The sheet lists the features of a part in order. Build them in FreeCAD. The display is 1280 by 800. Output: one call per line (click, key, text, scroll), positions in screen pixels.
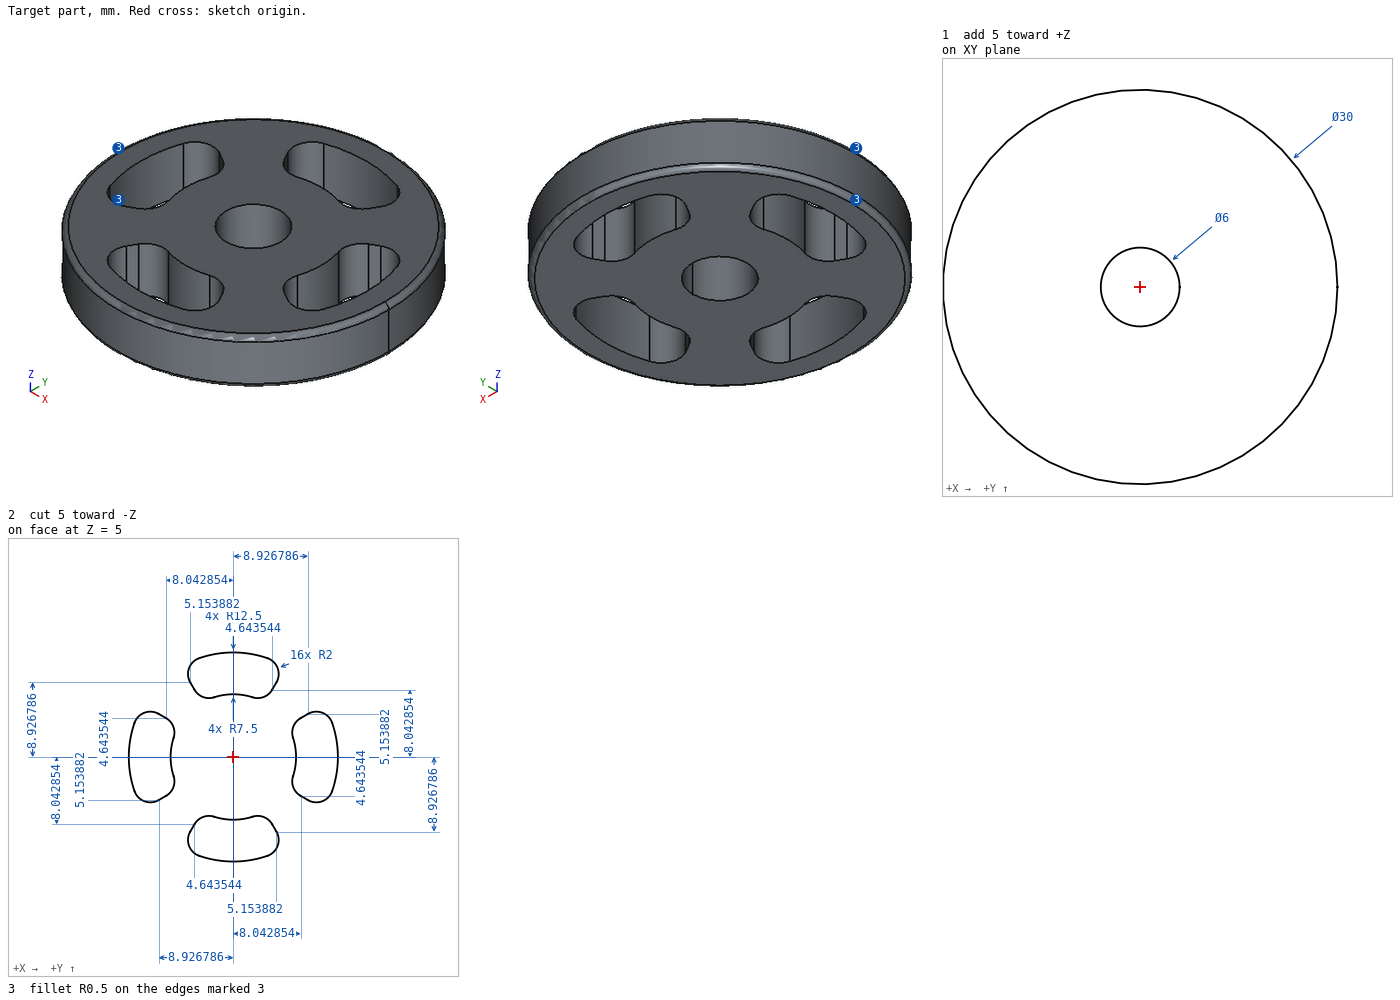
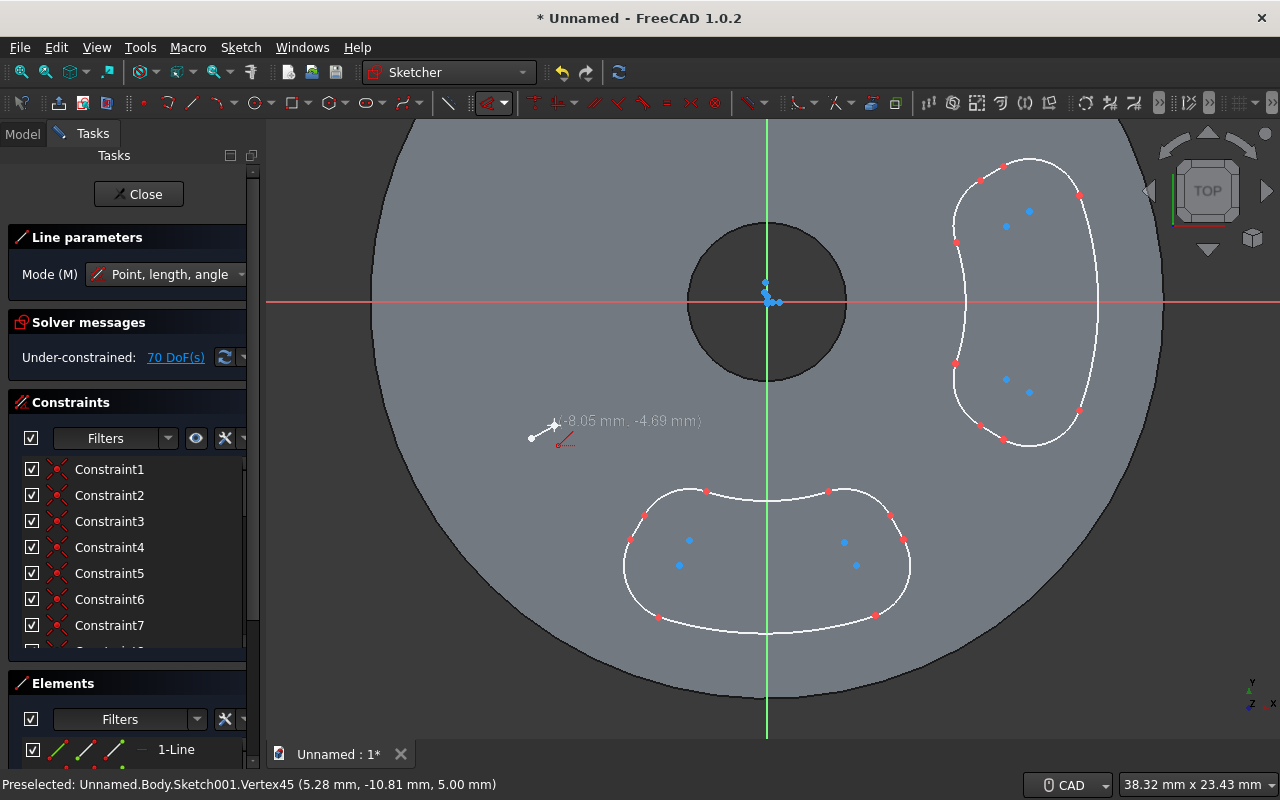
click(554, 179)
click(531, 166)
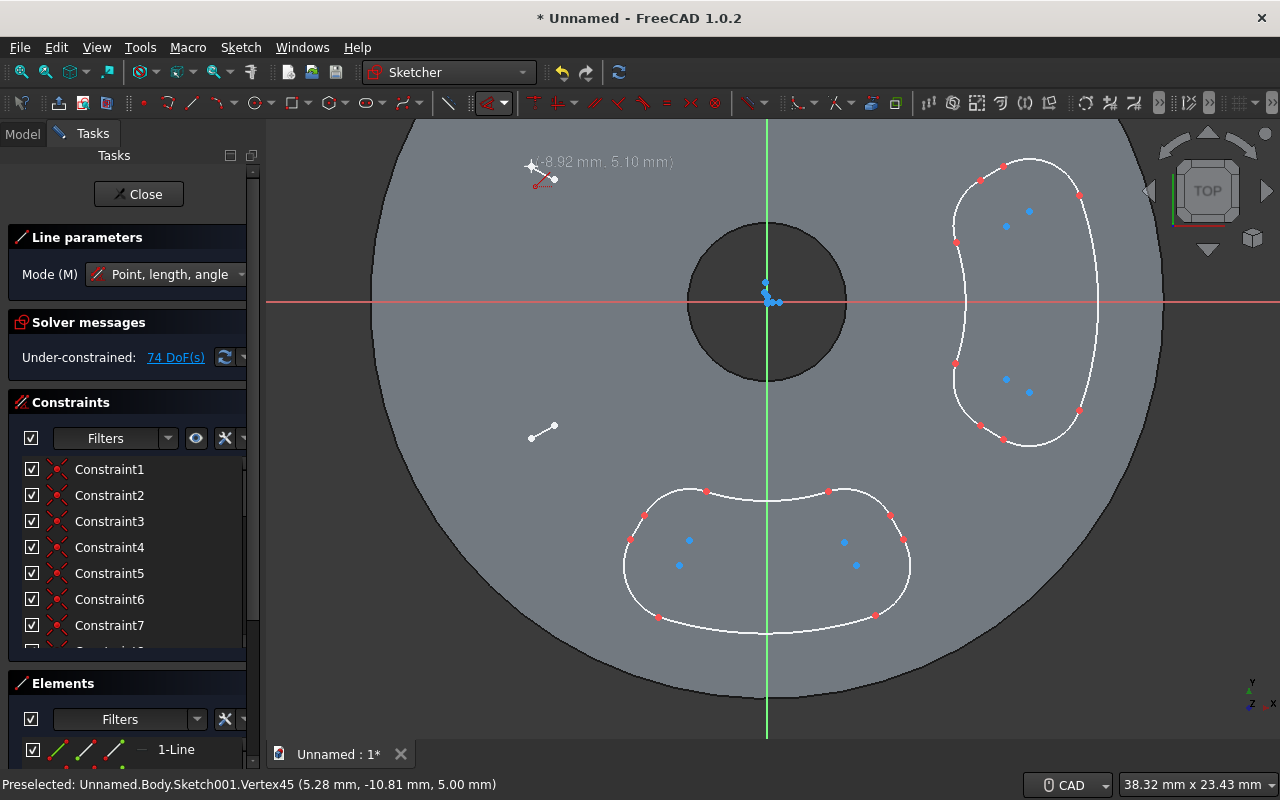
click(218, 104)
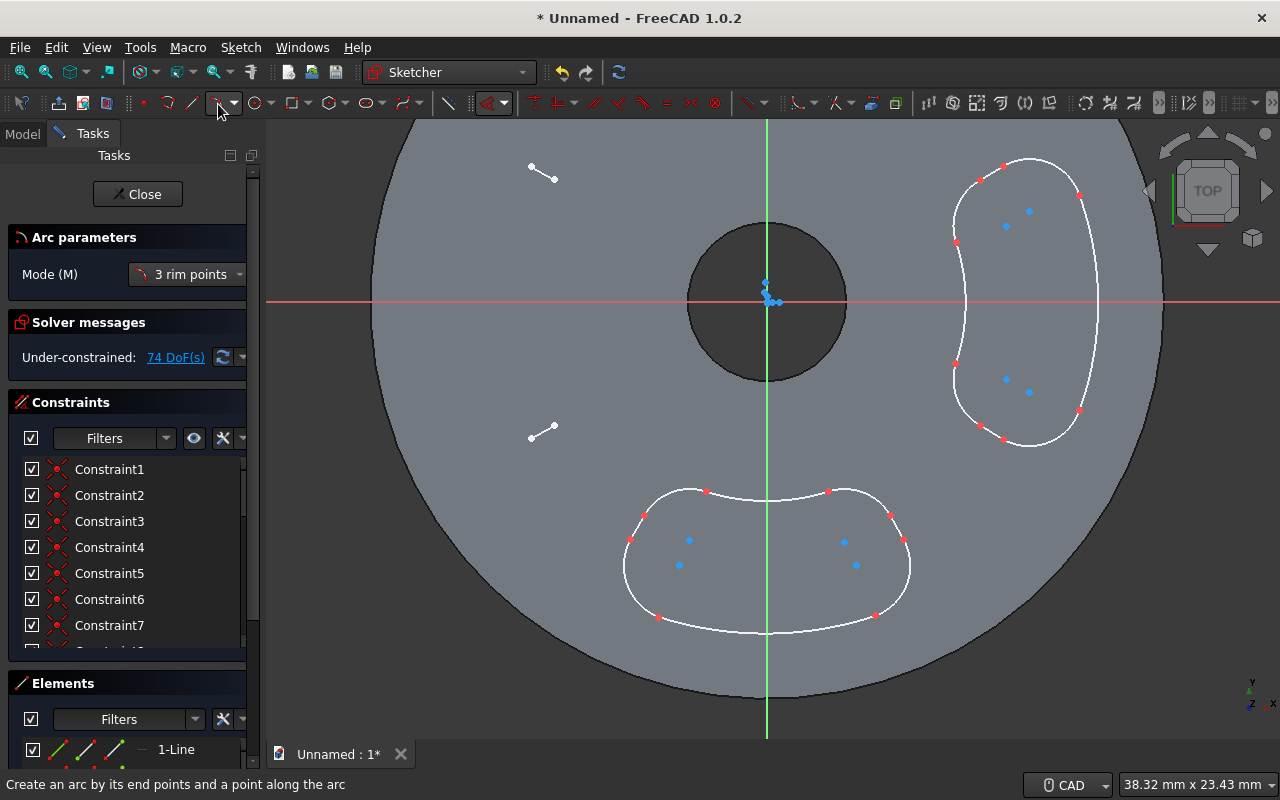
click(554, 426)
click(578, 363)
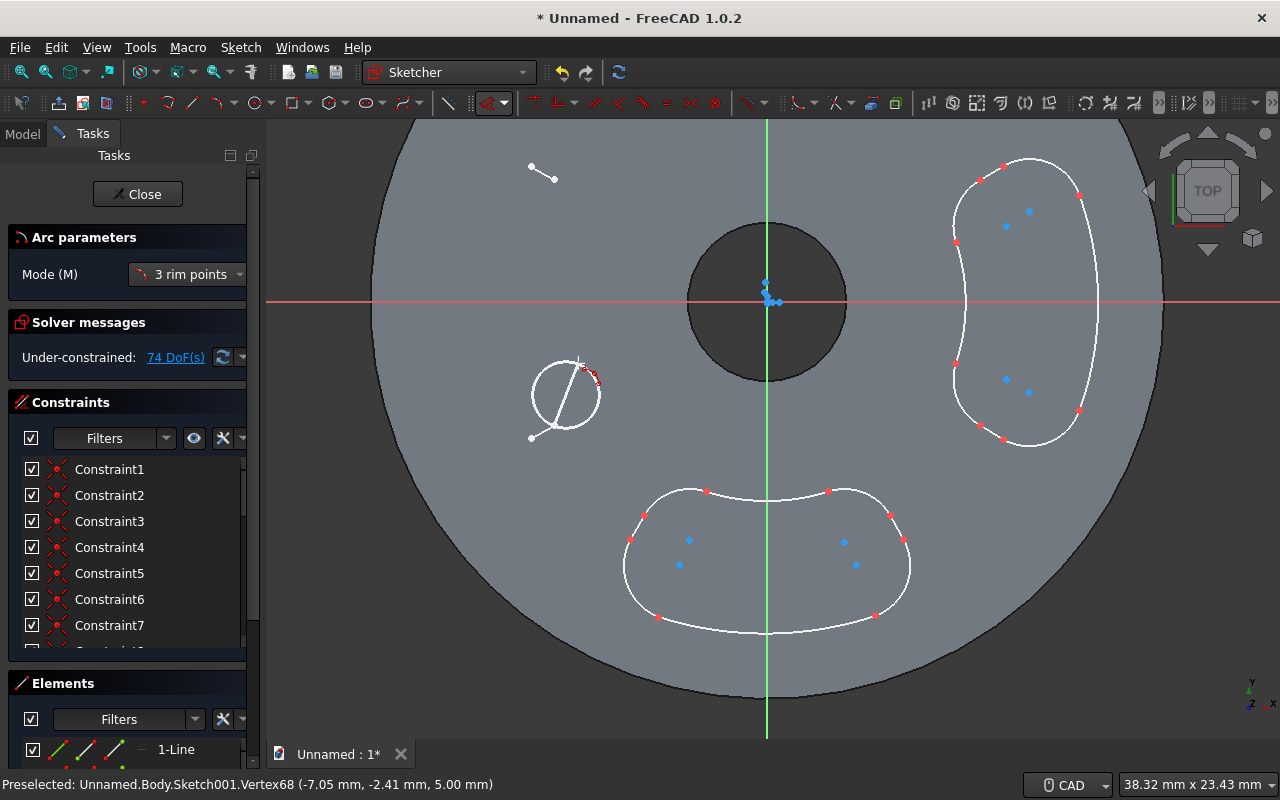
scroll(577, 398, up, 2)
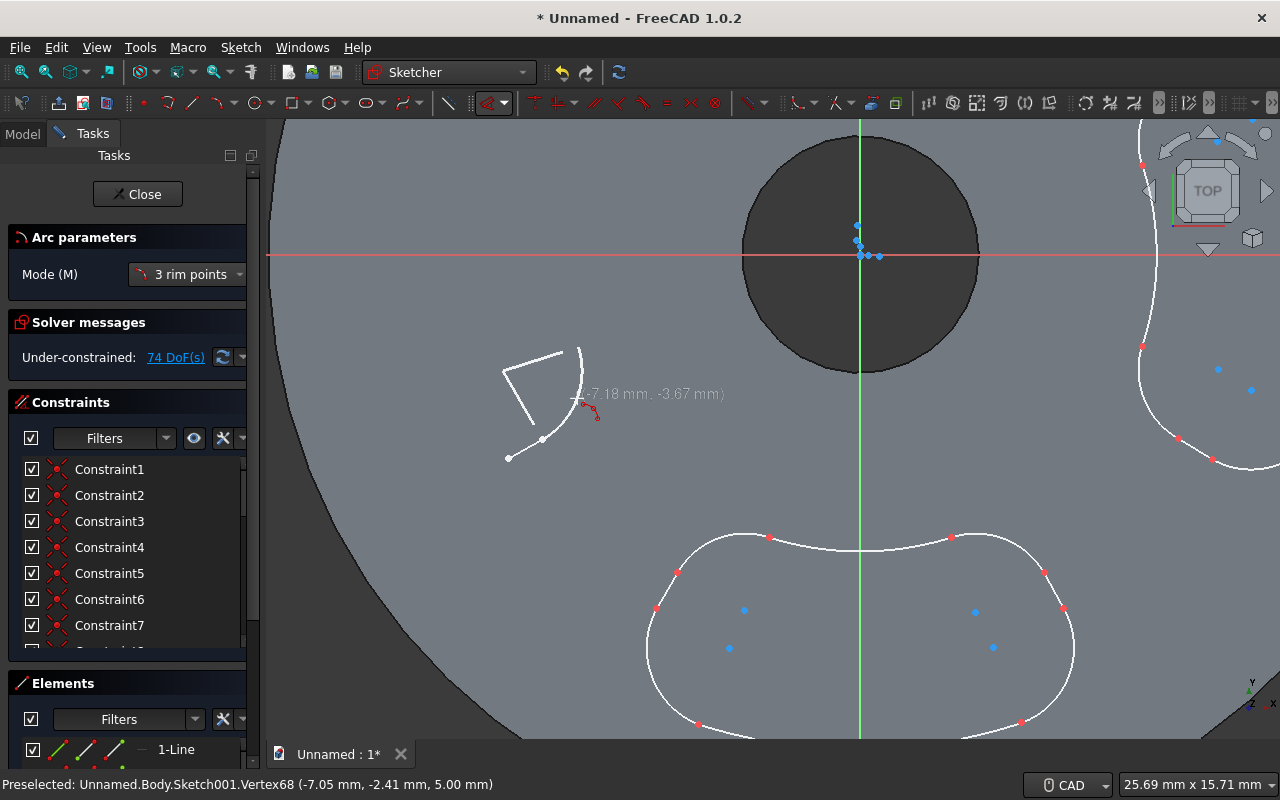
click(577, 398)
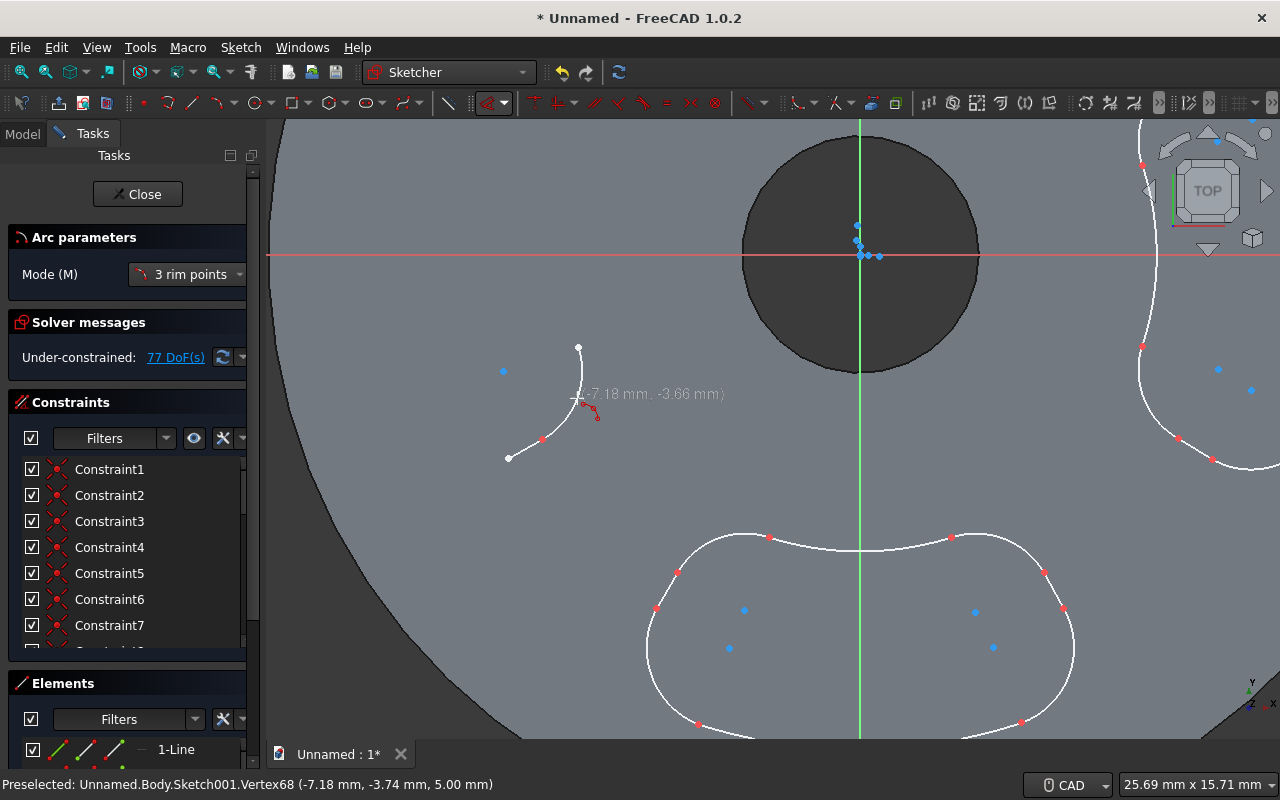
click(578, 347)
click(579, 164)
click(565, 236)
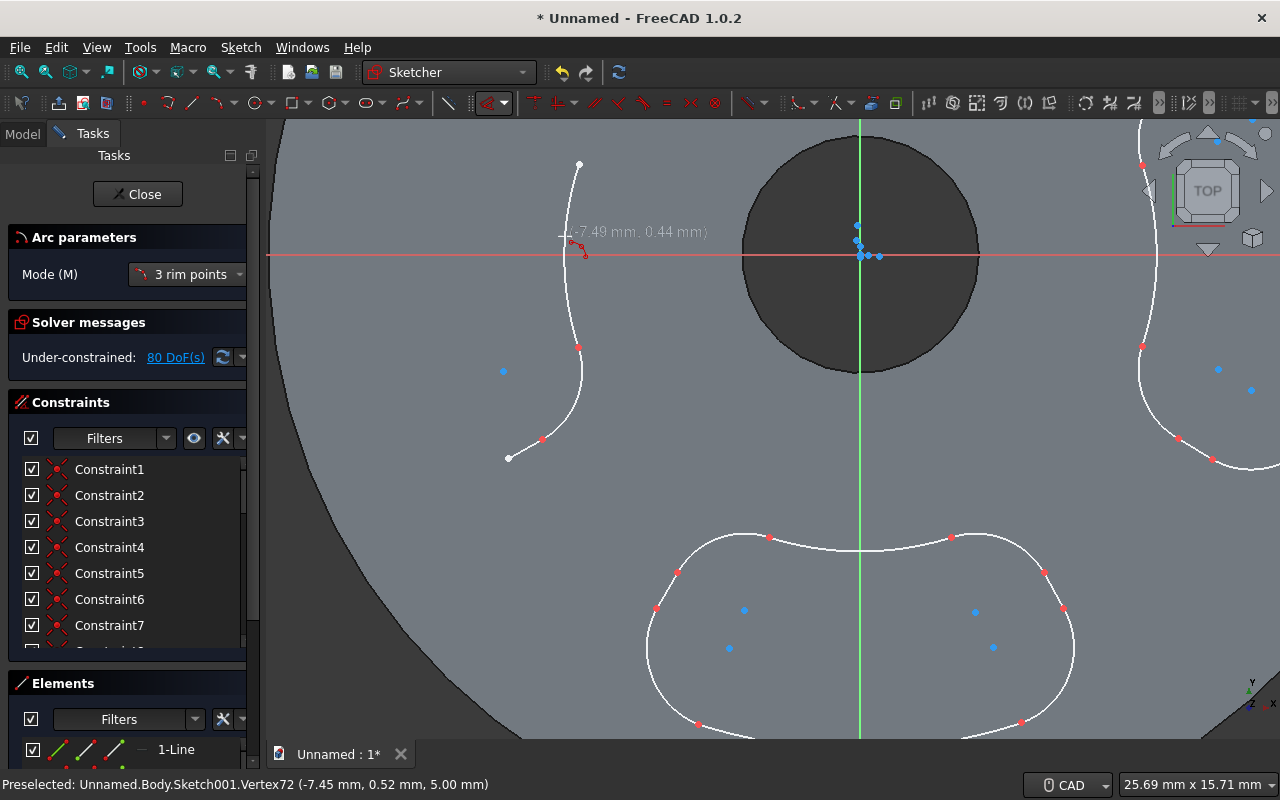
click(579, 165)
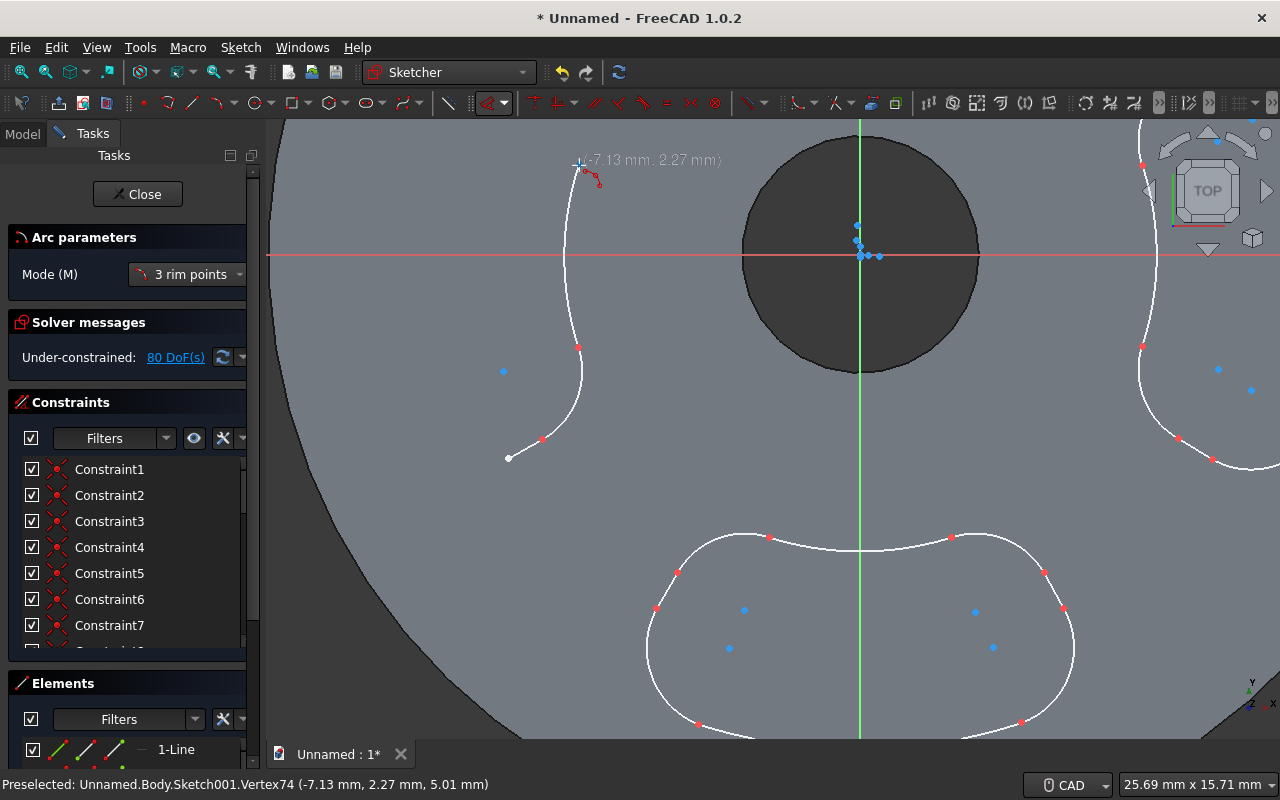
scroll(614, 531, down, 5)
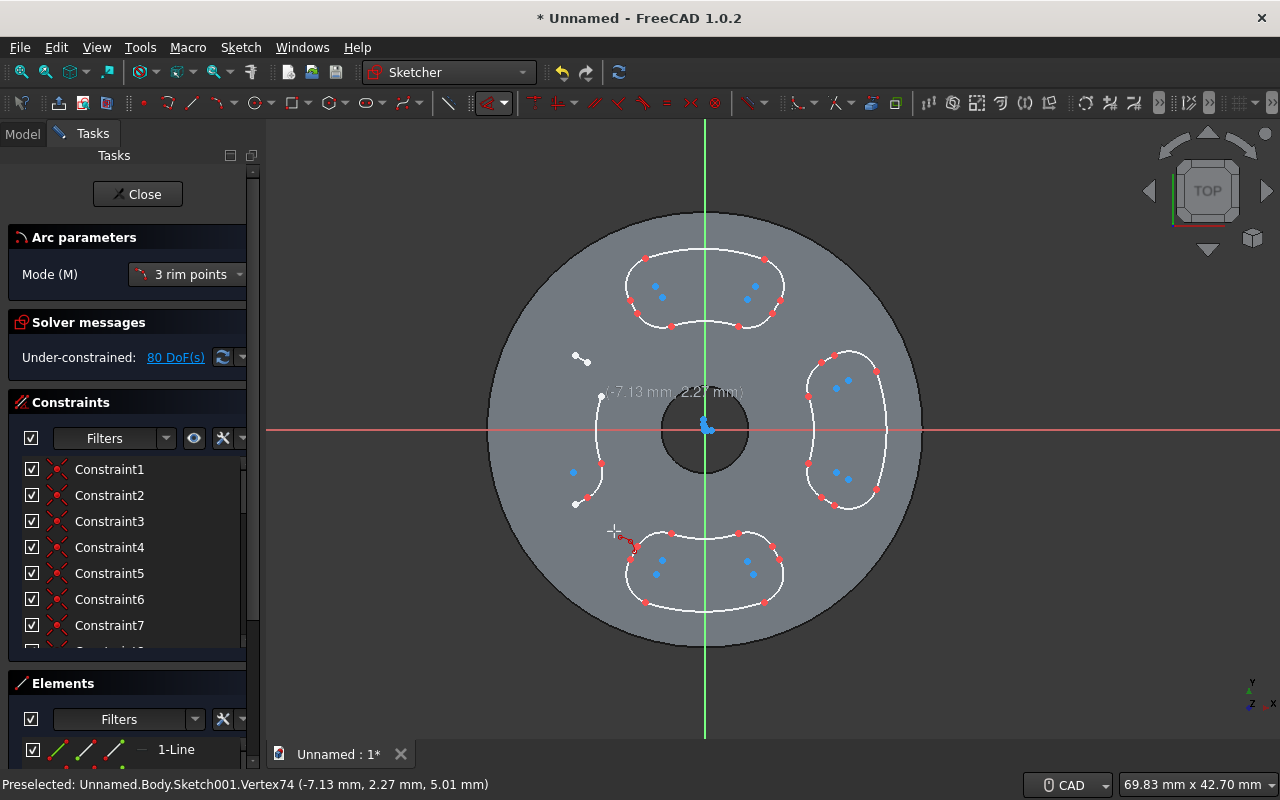
scroll(588, 362, up, 4)